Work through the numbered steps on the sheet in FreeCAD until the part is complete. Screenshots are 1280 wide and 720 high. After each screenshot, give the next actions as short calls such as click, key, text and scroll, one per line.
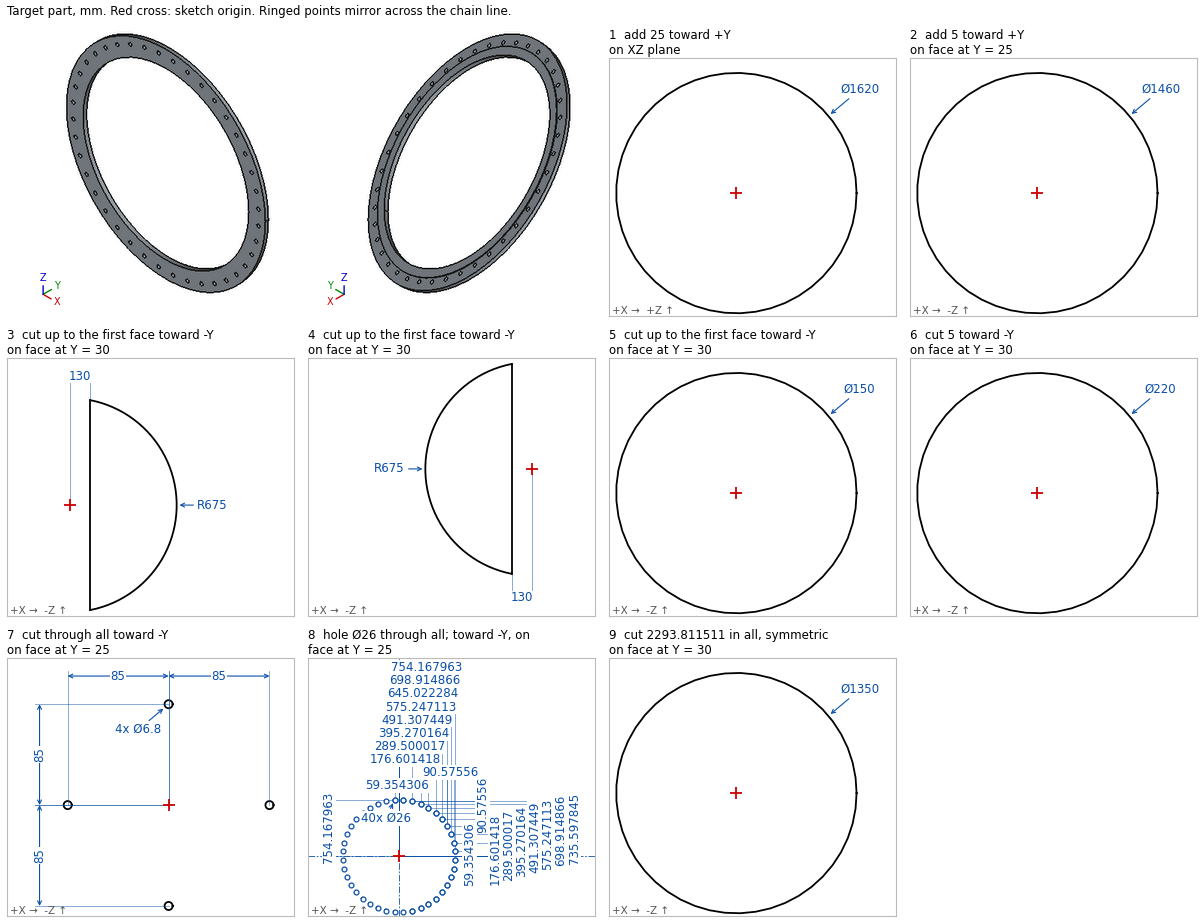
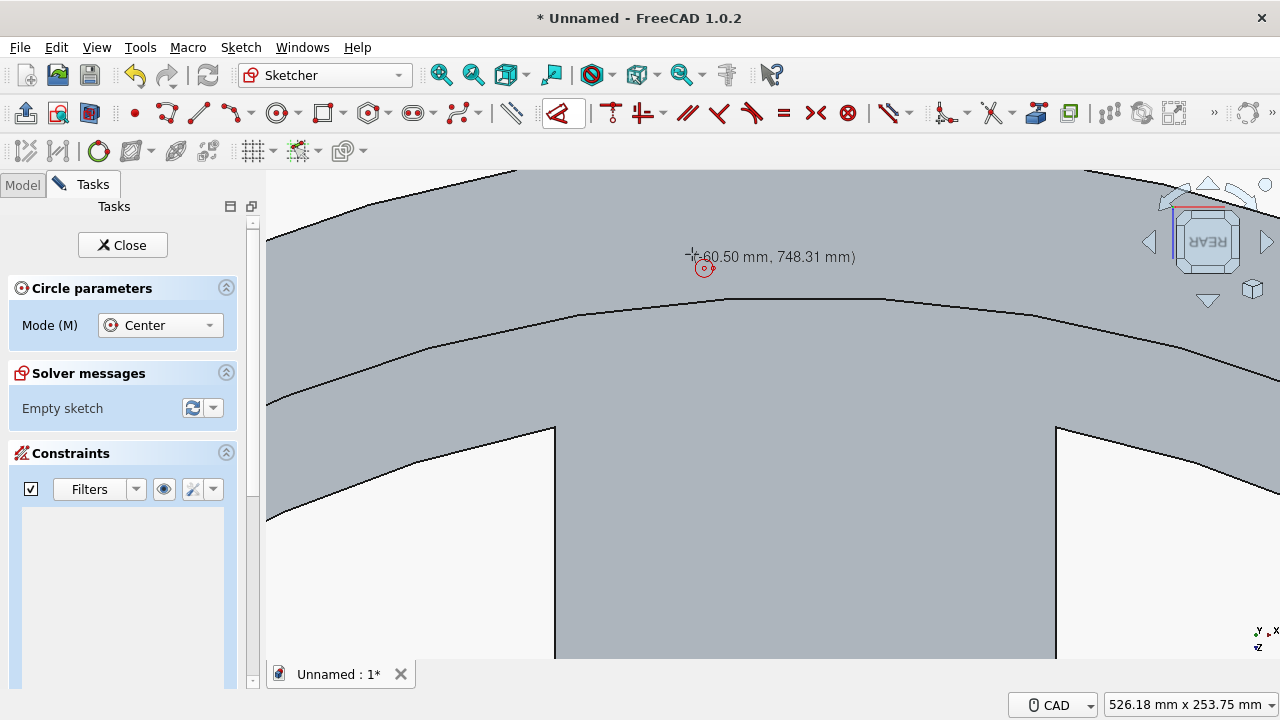
scroll(692, 254, down, 11)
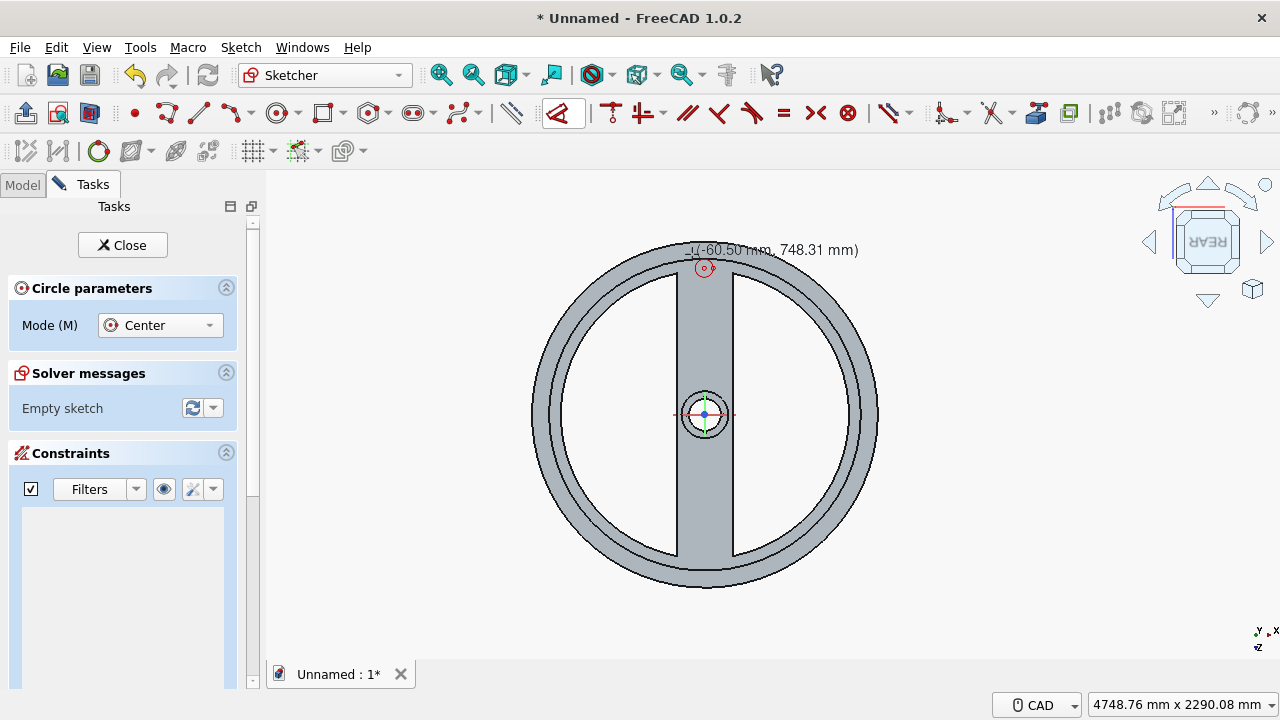
scroll(692, 254, up, 2)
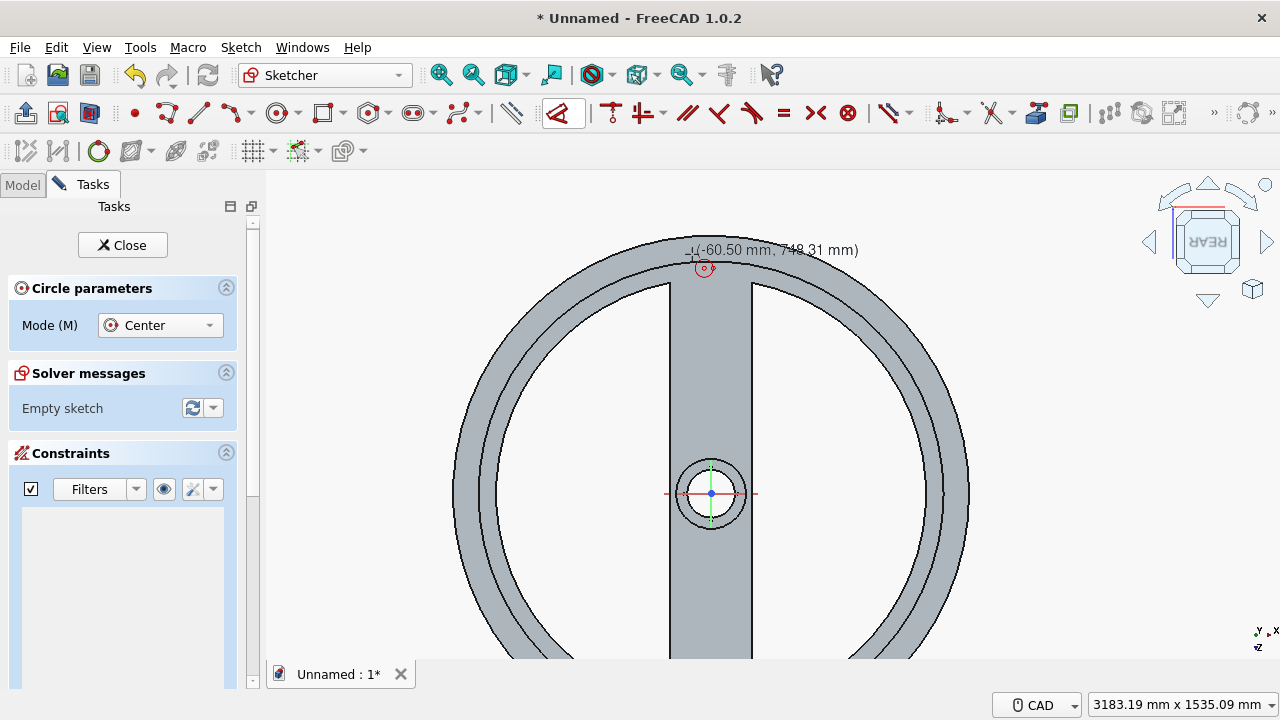
click(692, 254)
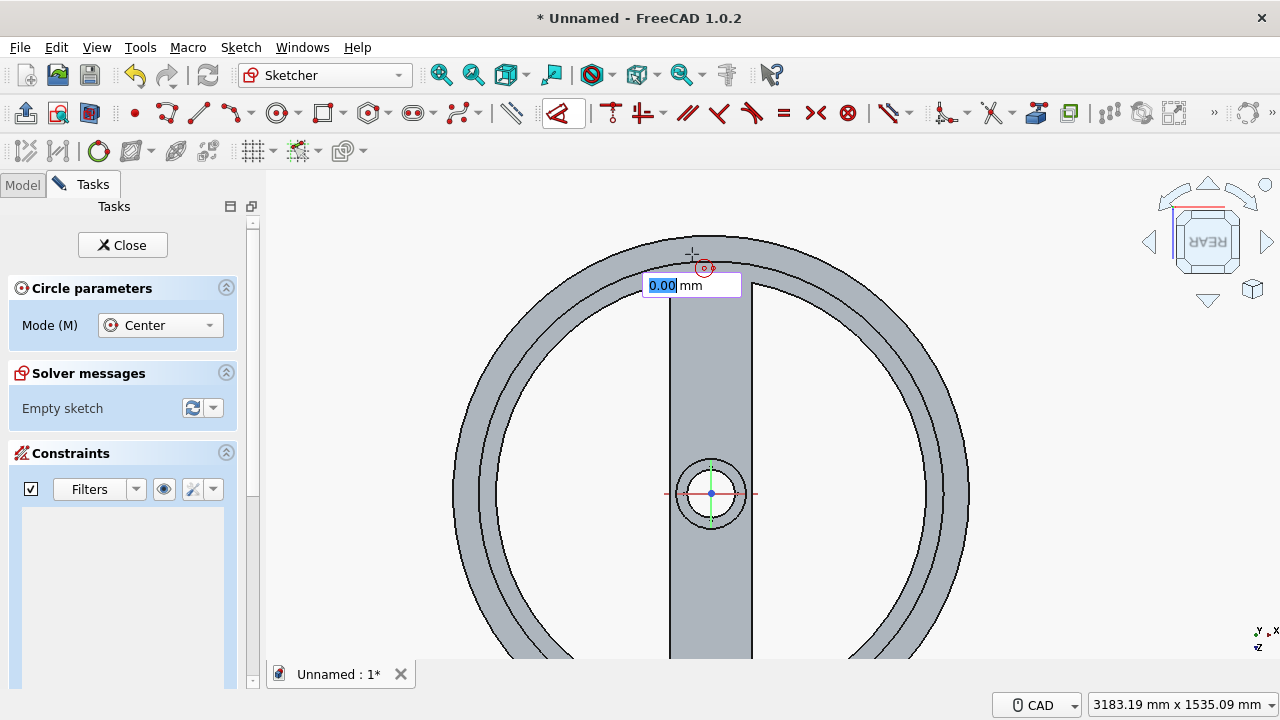
scroll(695, 251, up, 7)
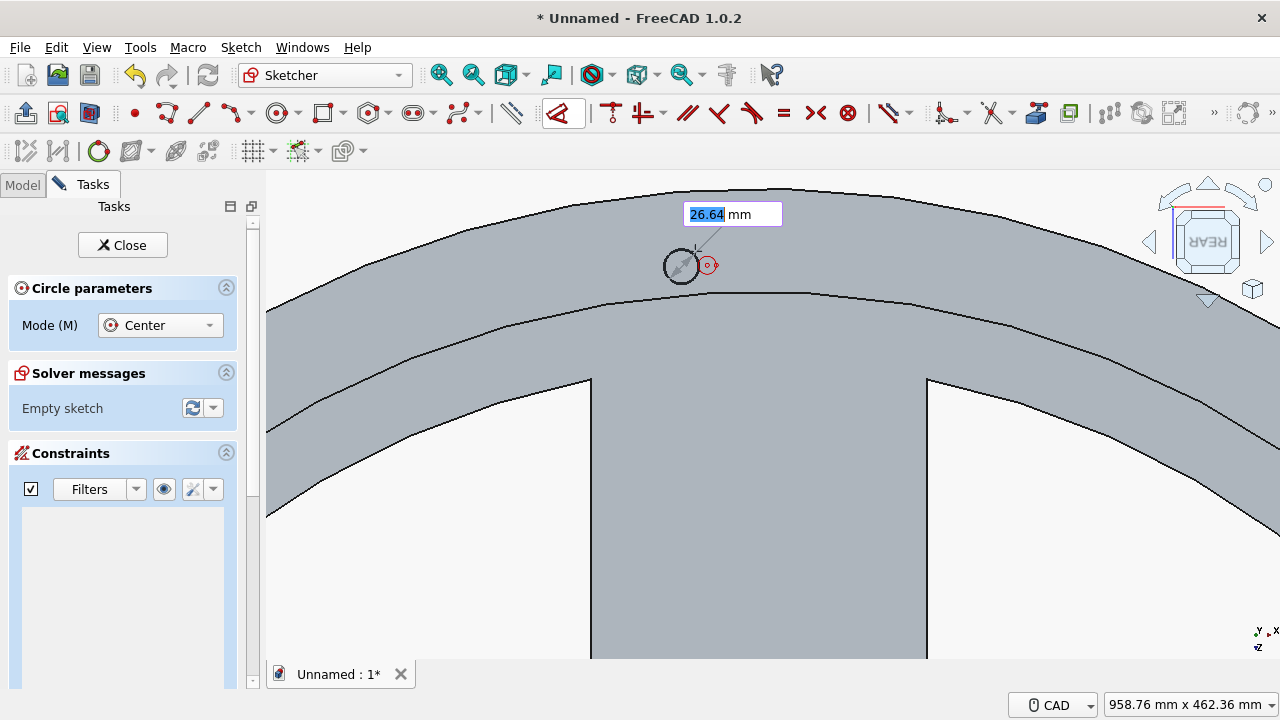
click(694, 249)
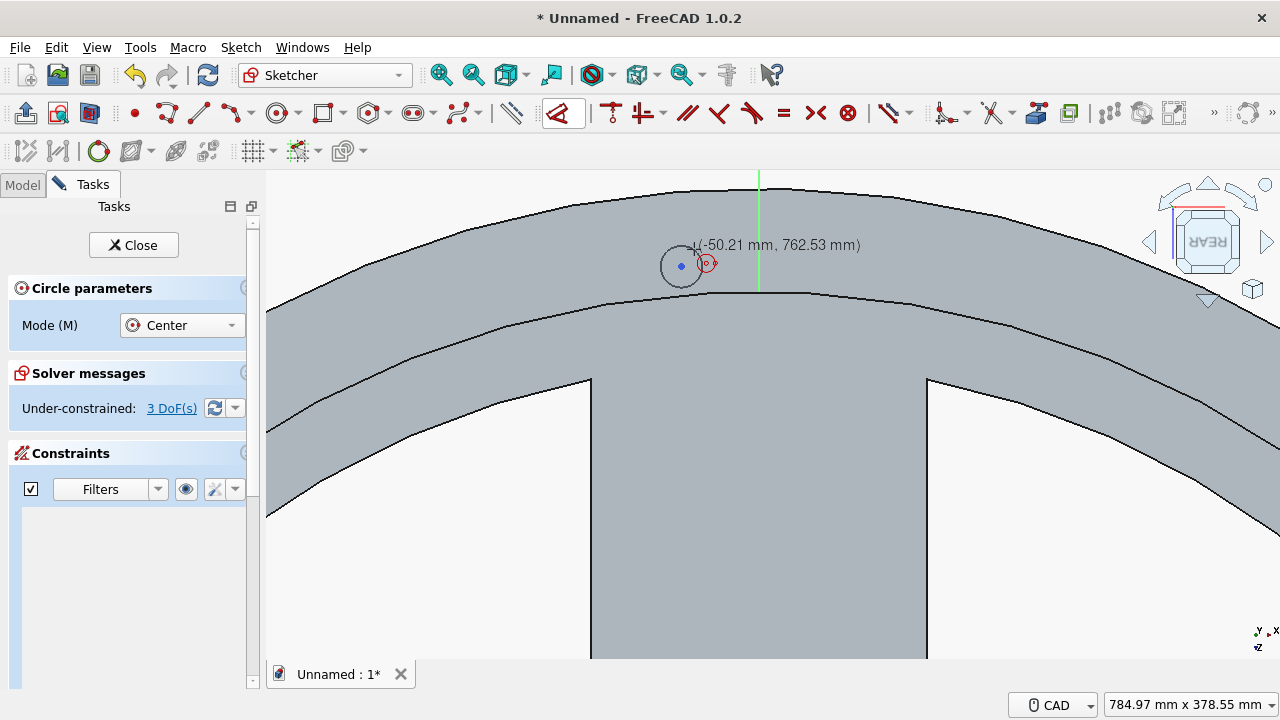
scroll(836, 261, up, 2)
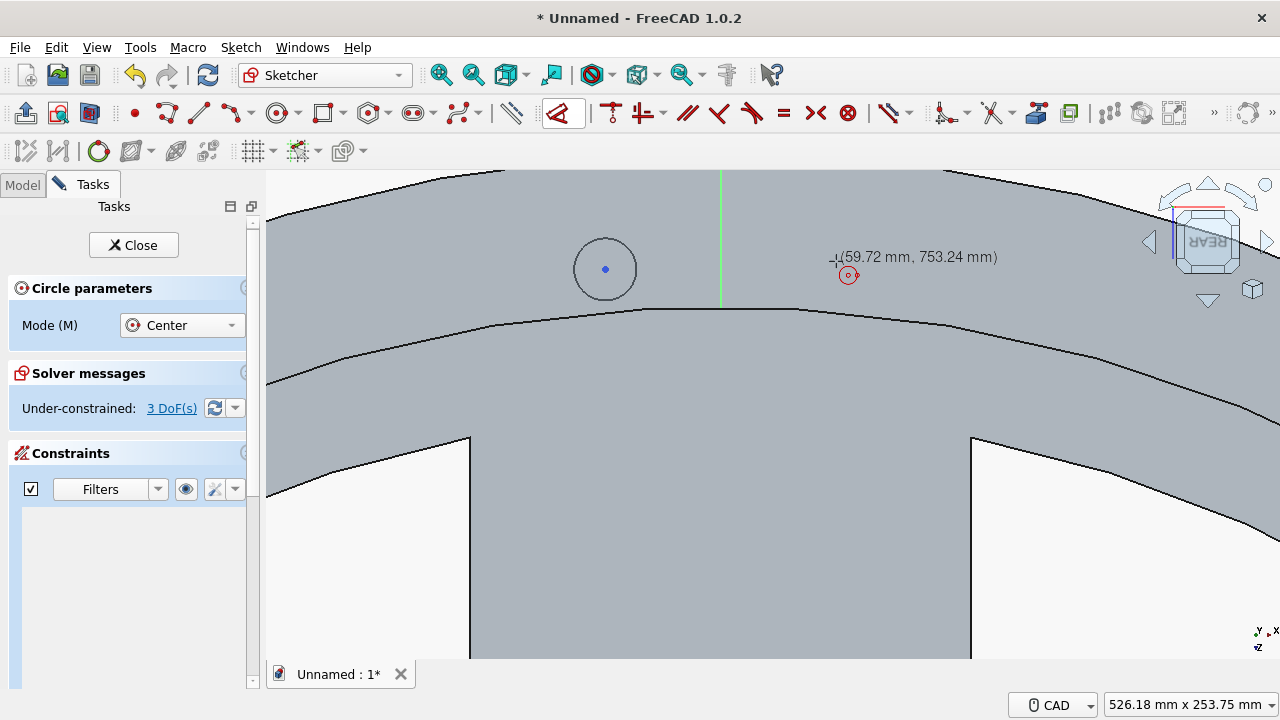
scroll(702, 253, down, 11)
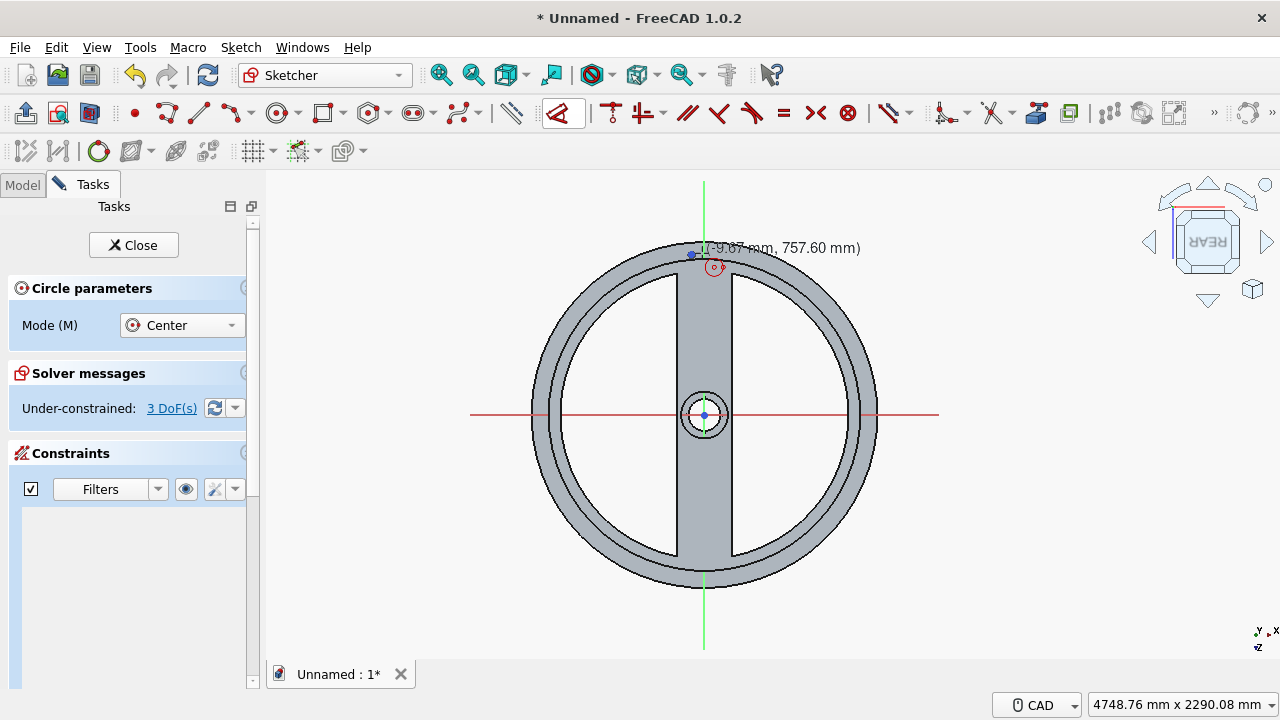
scroll(717, 254, up, 2)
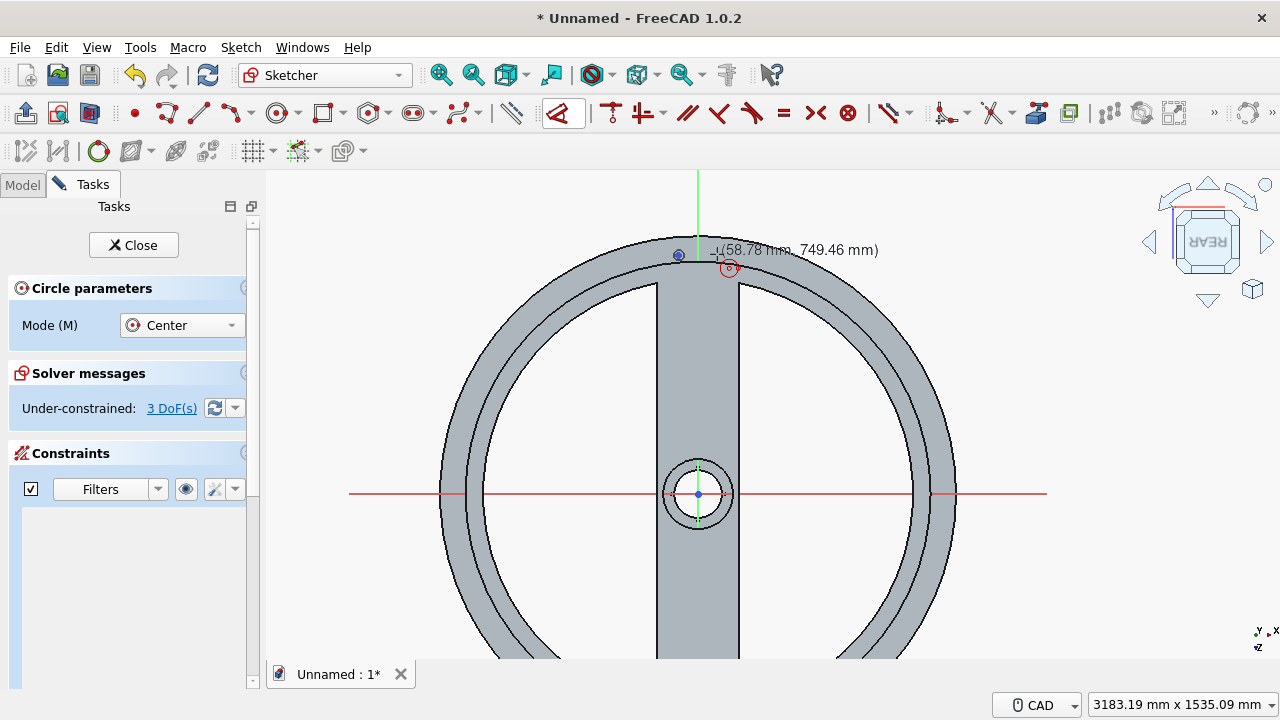
click(717, 254)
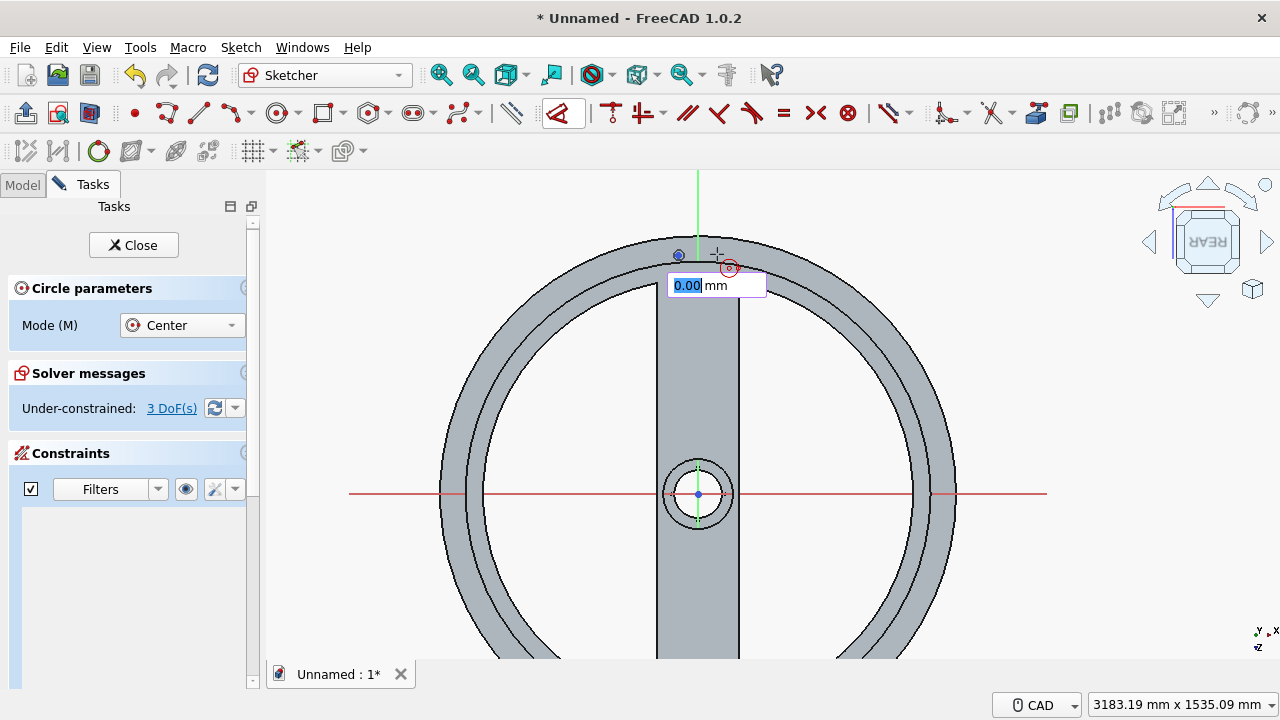
scroll(720, 251, up, 7)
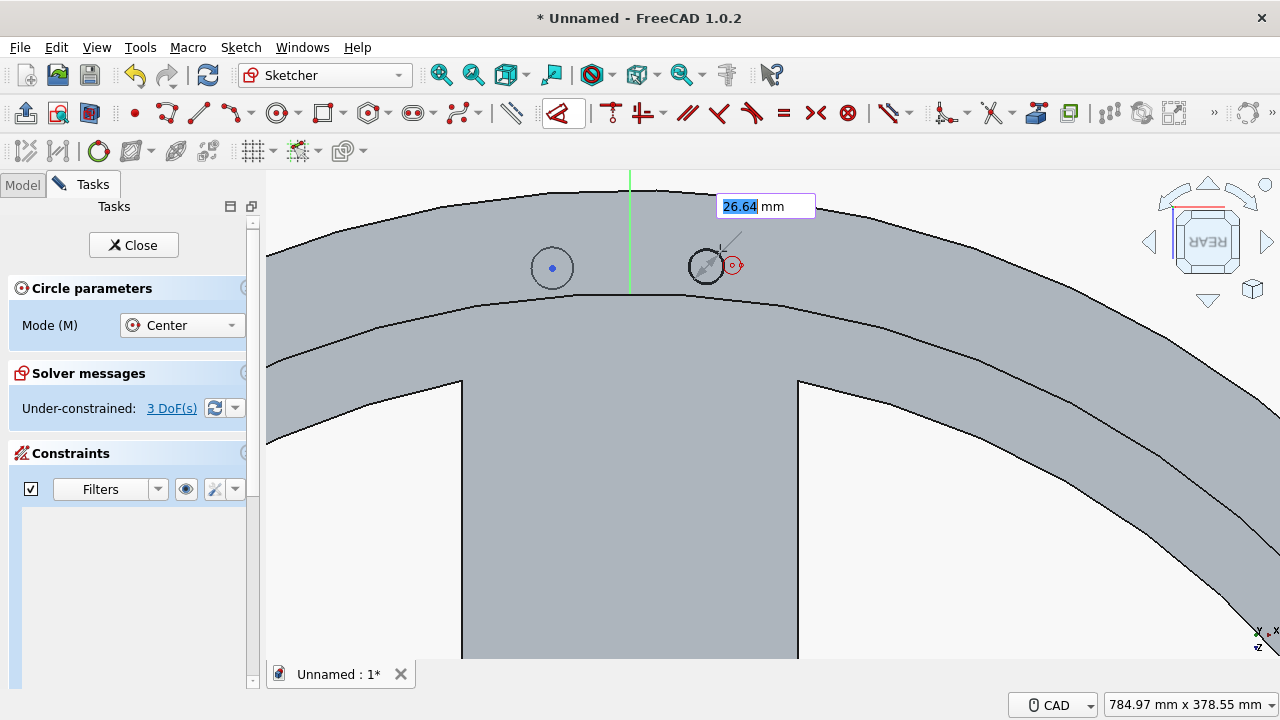
click(718, 250)